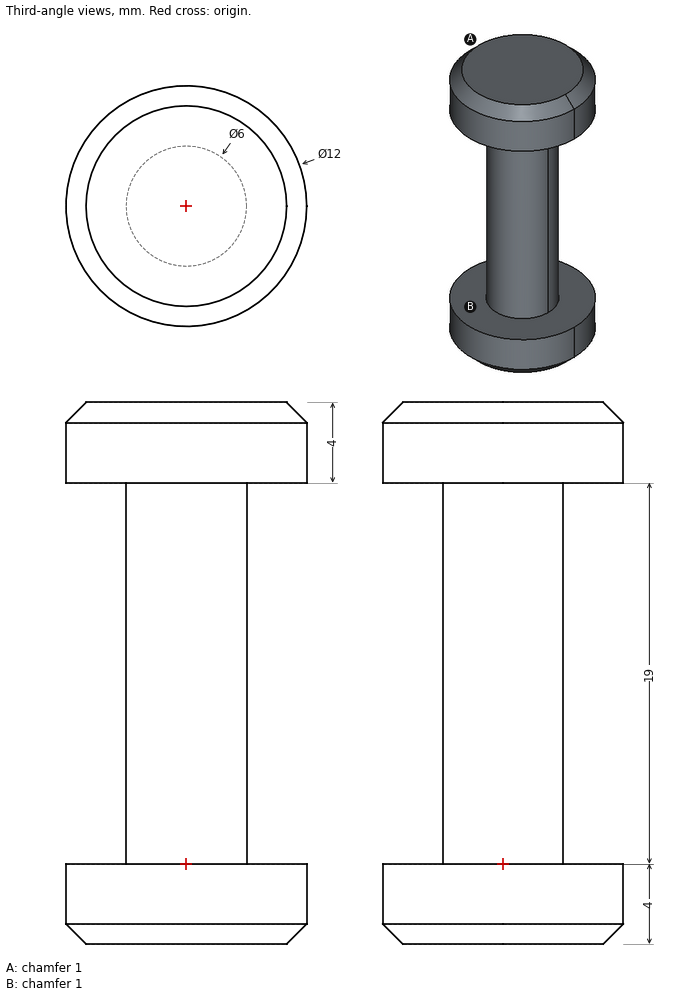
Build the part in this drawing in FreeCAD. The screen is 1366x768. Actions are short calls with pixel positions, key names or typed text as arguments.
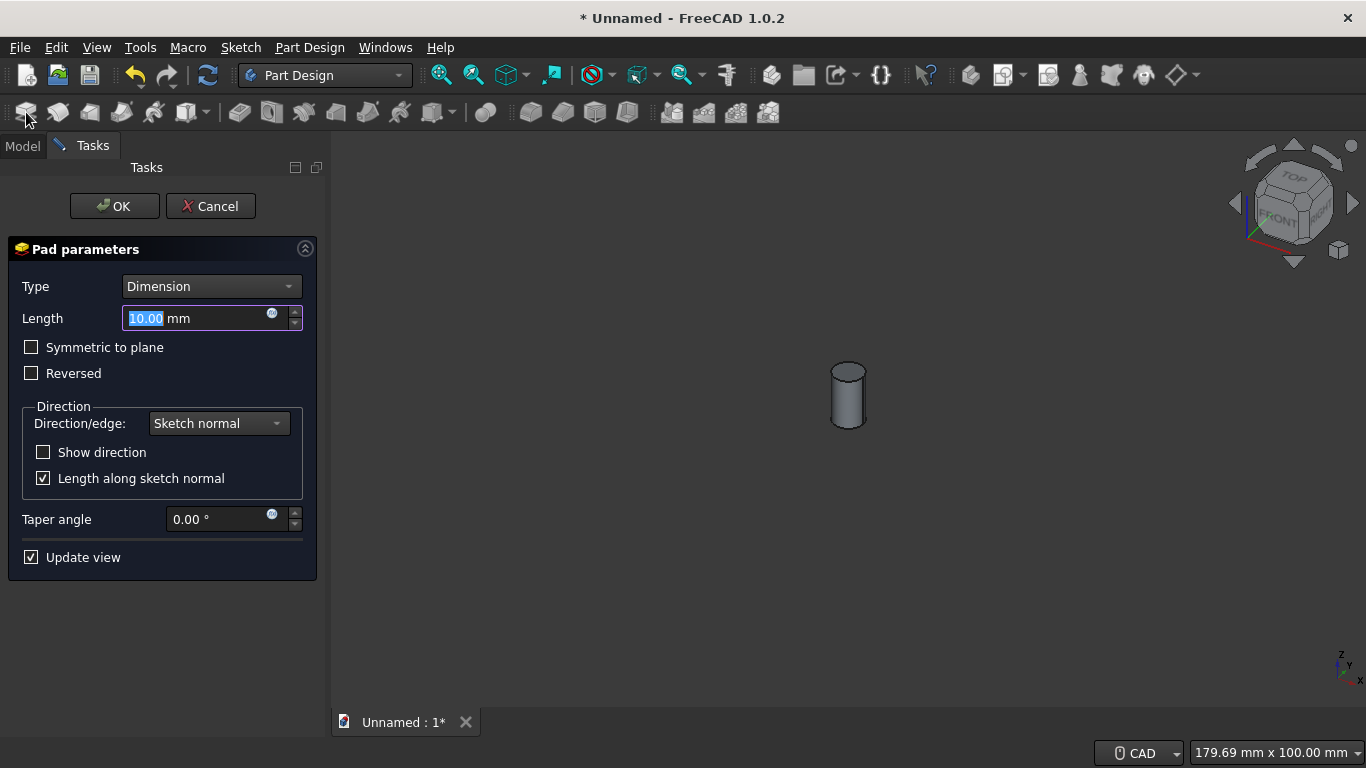
text(19)
key(Tab)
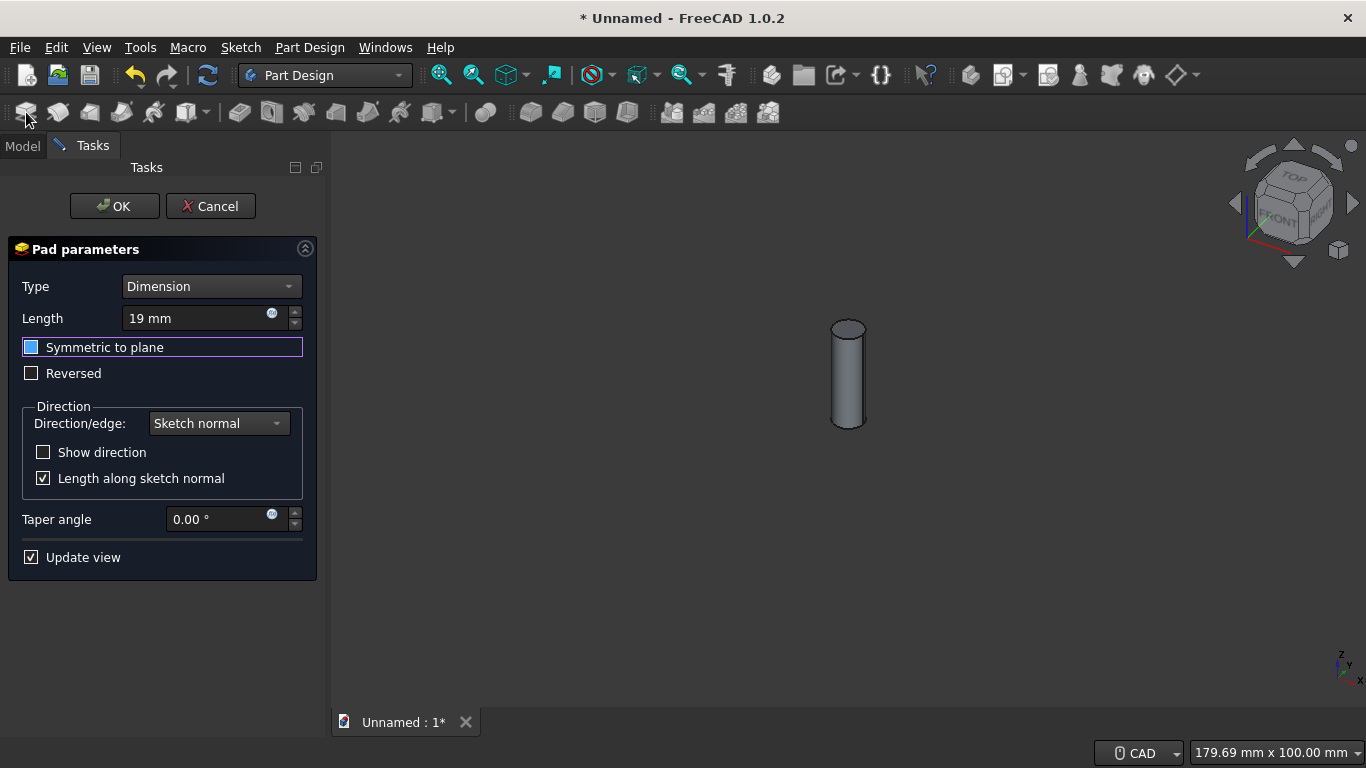
click(115, 206)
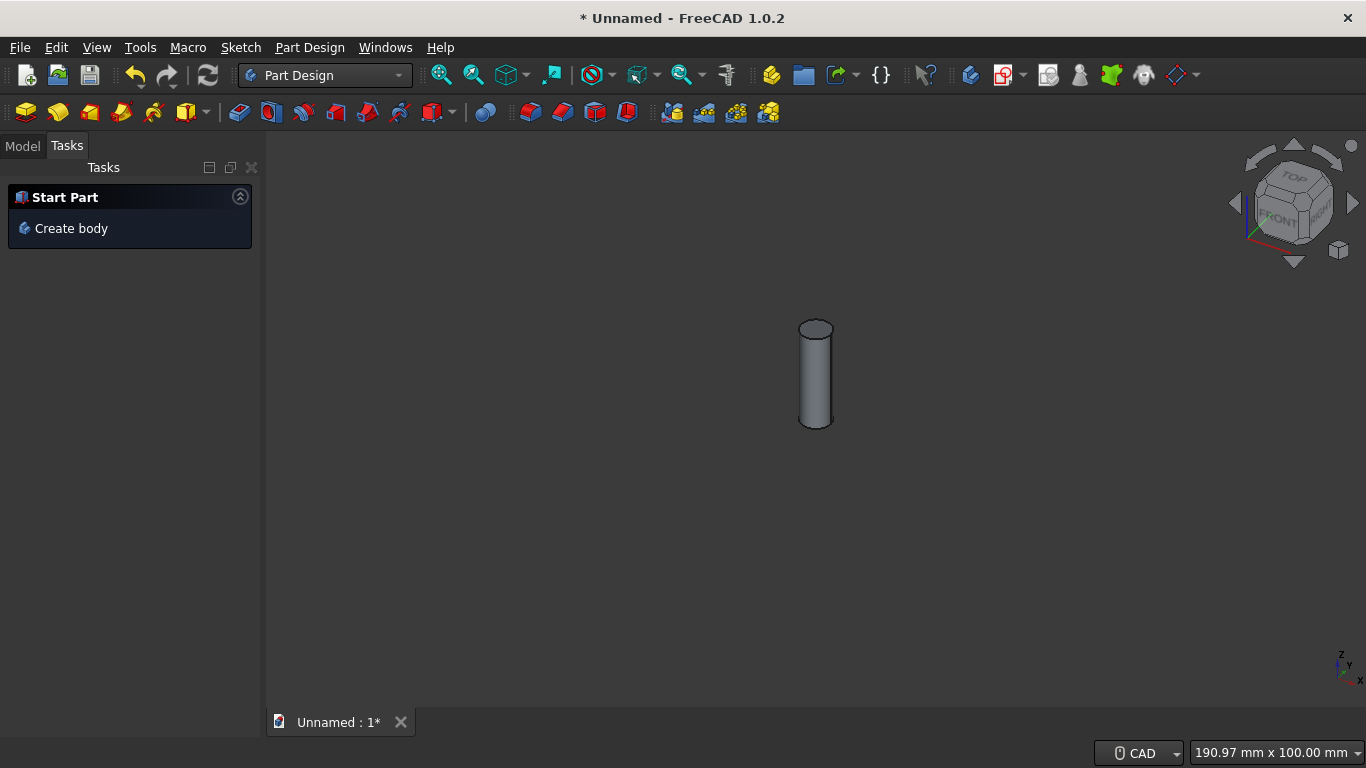
key(v)
key(f)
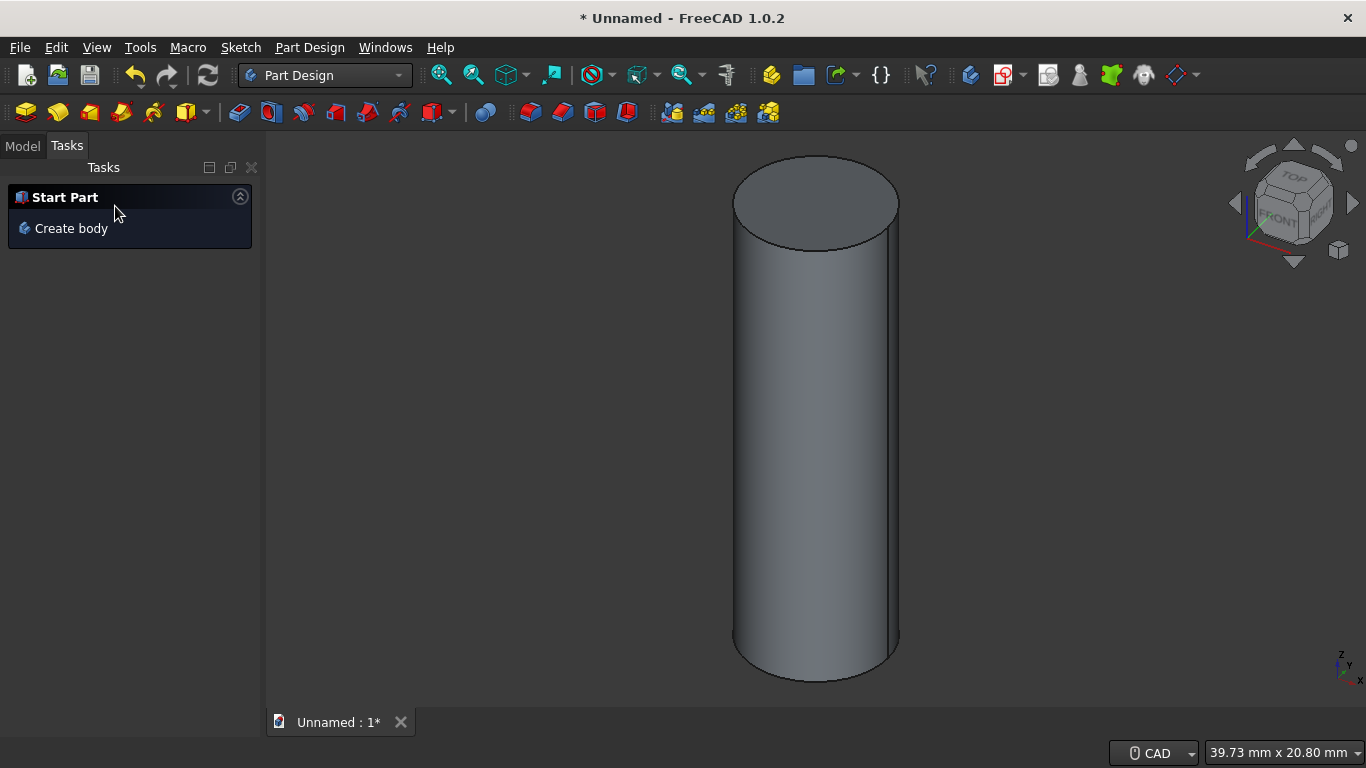
click(816, 203)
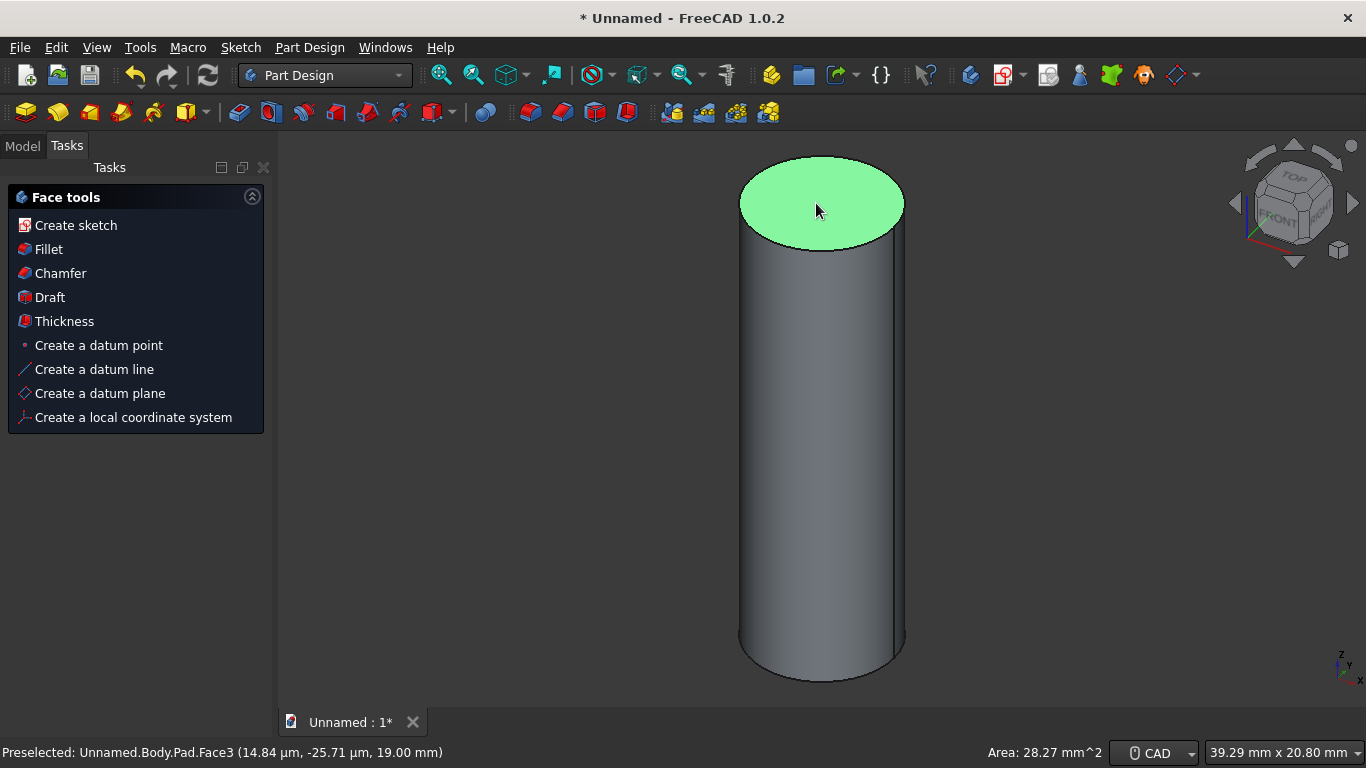
click(1004, 76)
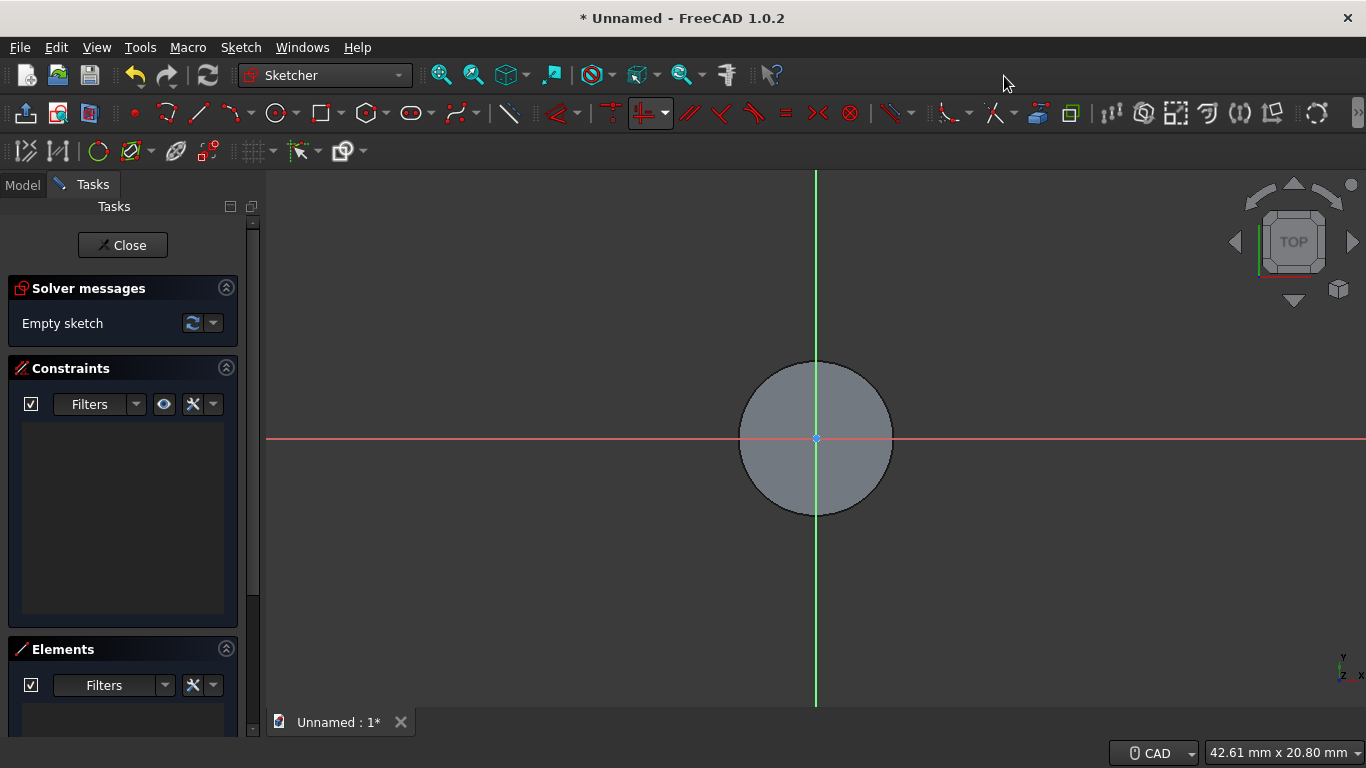
key(g)
key(c)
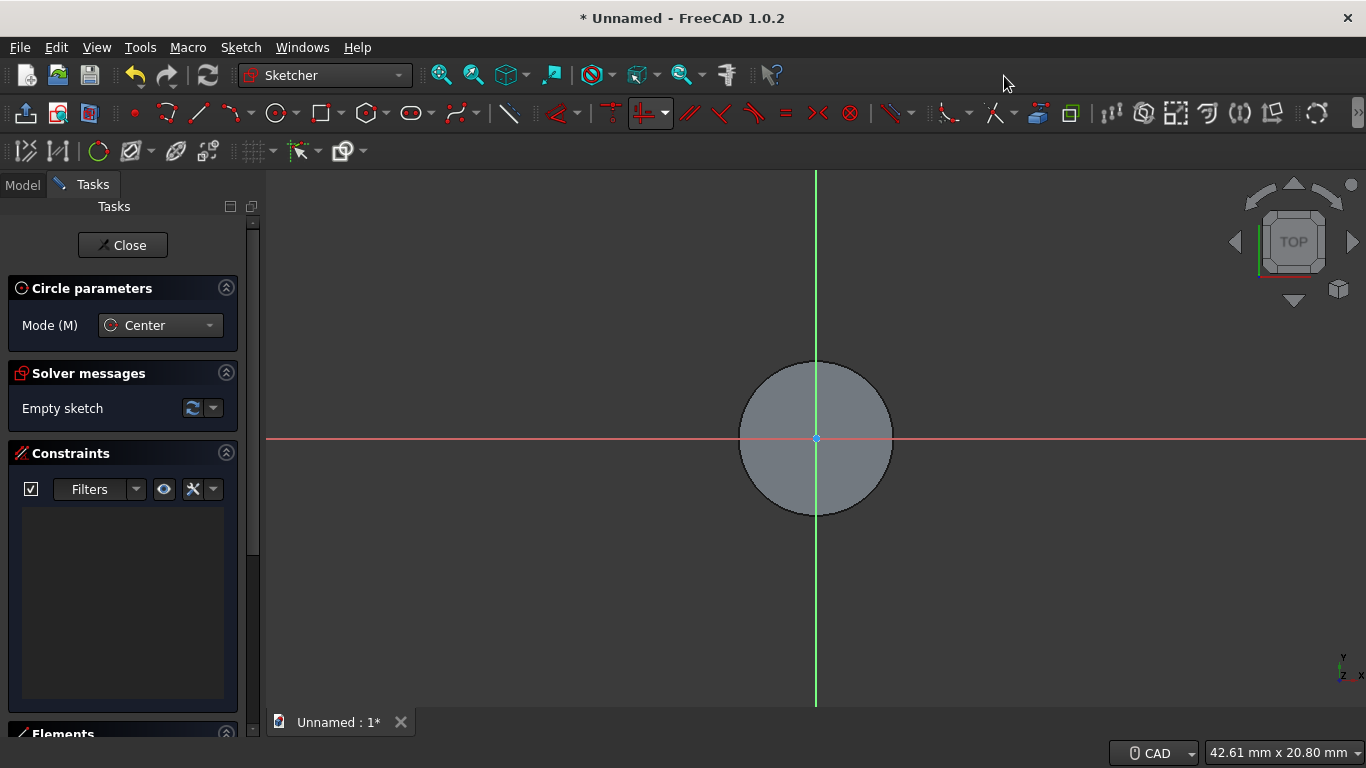
click(816, 438)
move(926, 329)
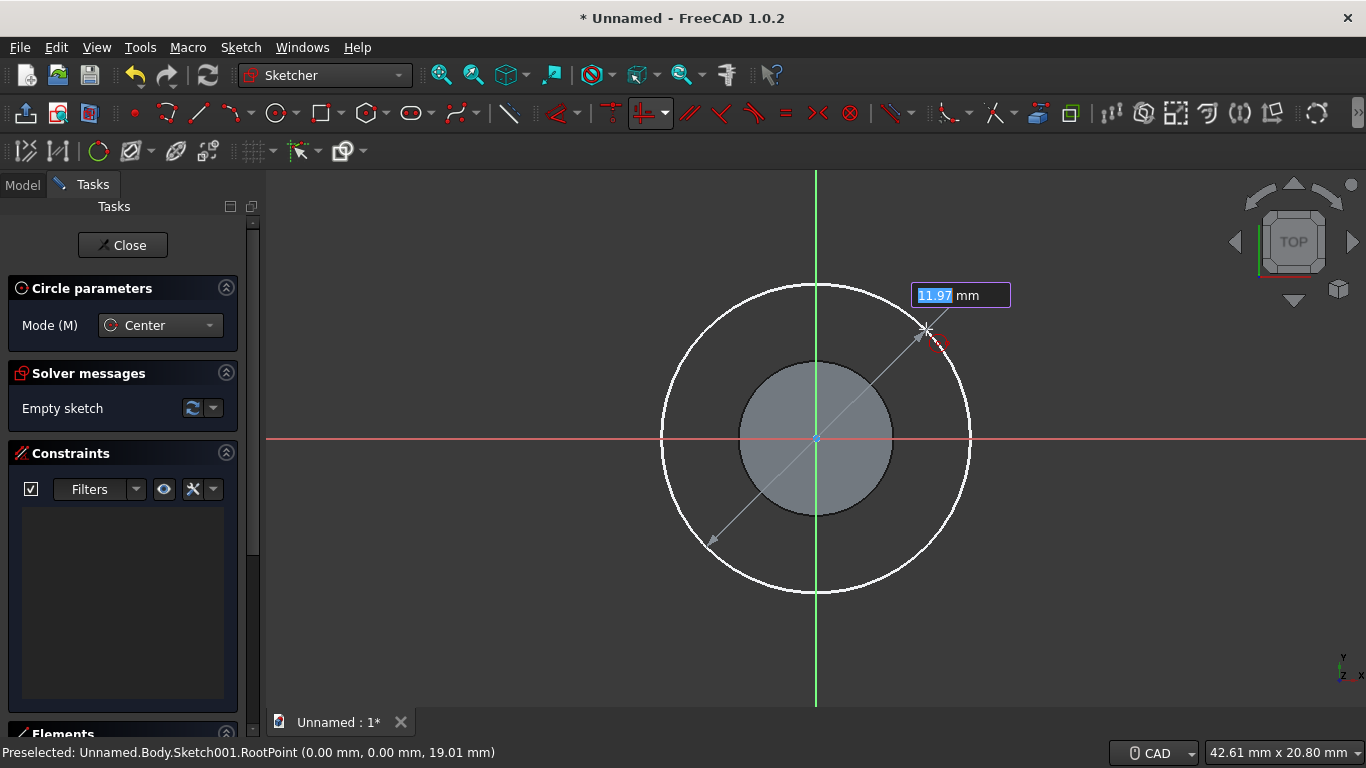
text(12)
key(Return)
key(Escape)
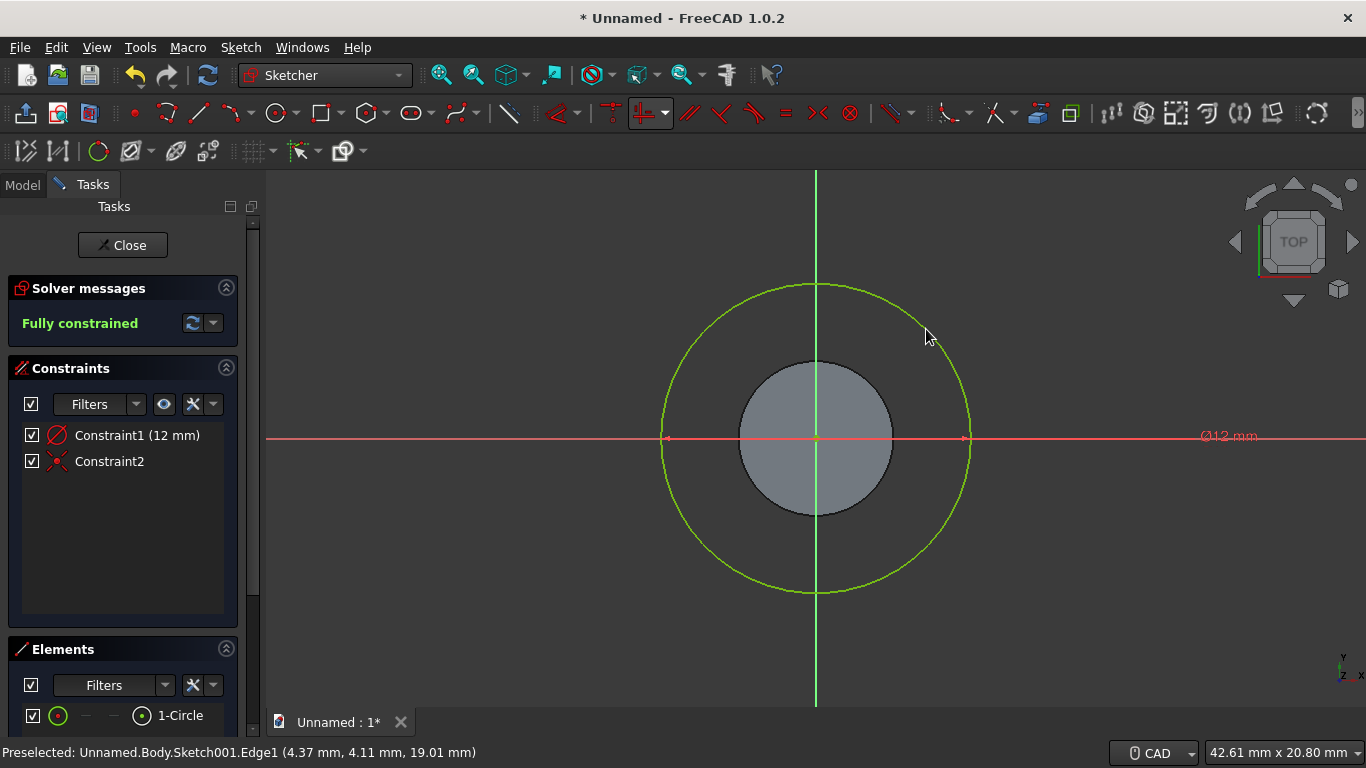
click(123, 245)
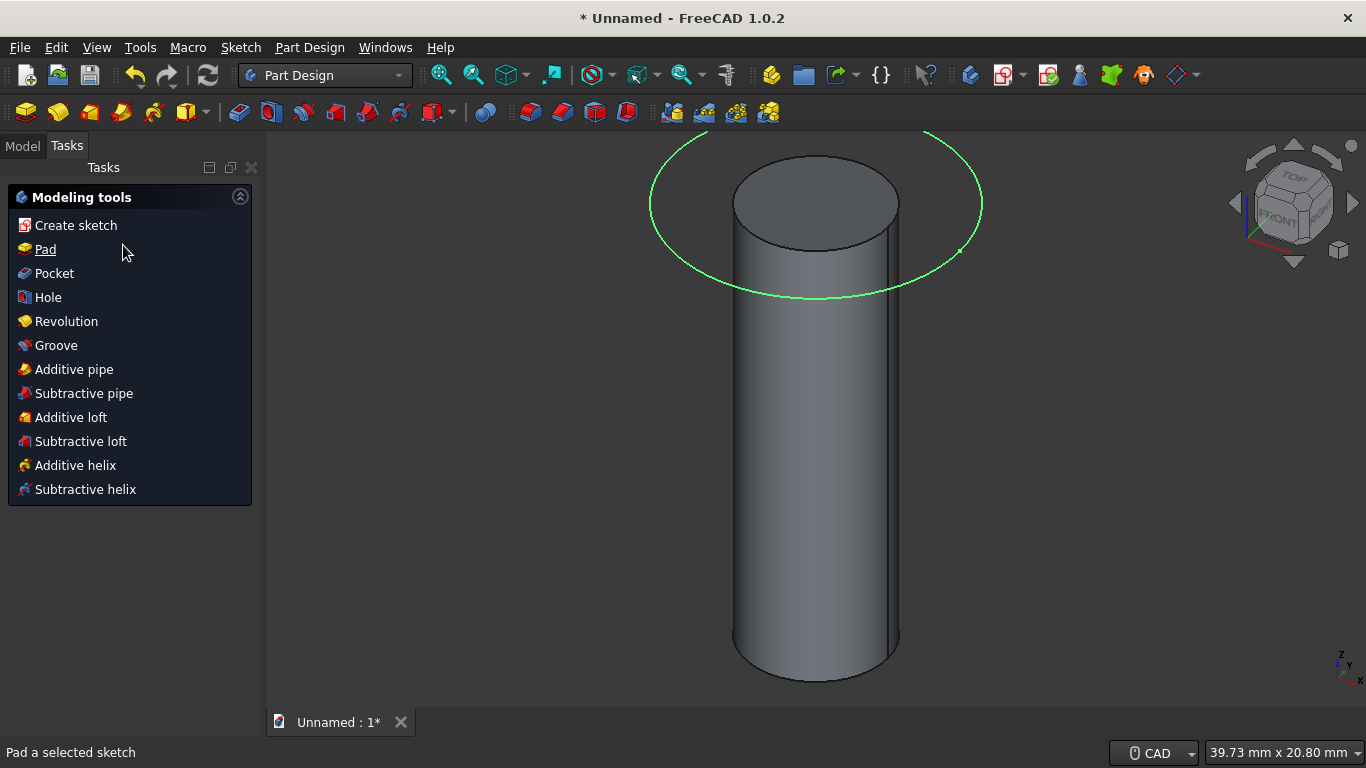
click(26, 112)